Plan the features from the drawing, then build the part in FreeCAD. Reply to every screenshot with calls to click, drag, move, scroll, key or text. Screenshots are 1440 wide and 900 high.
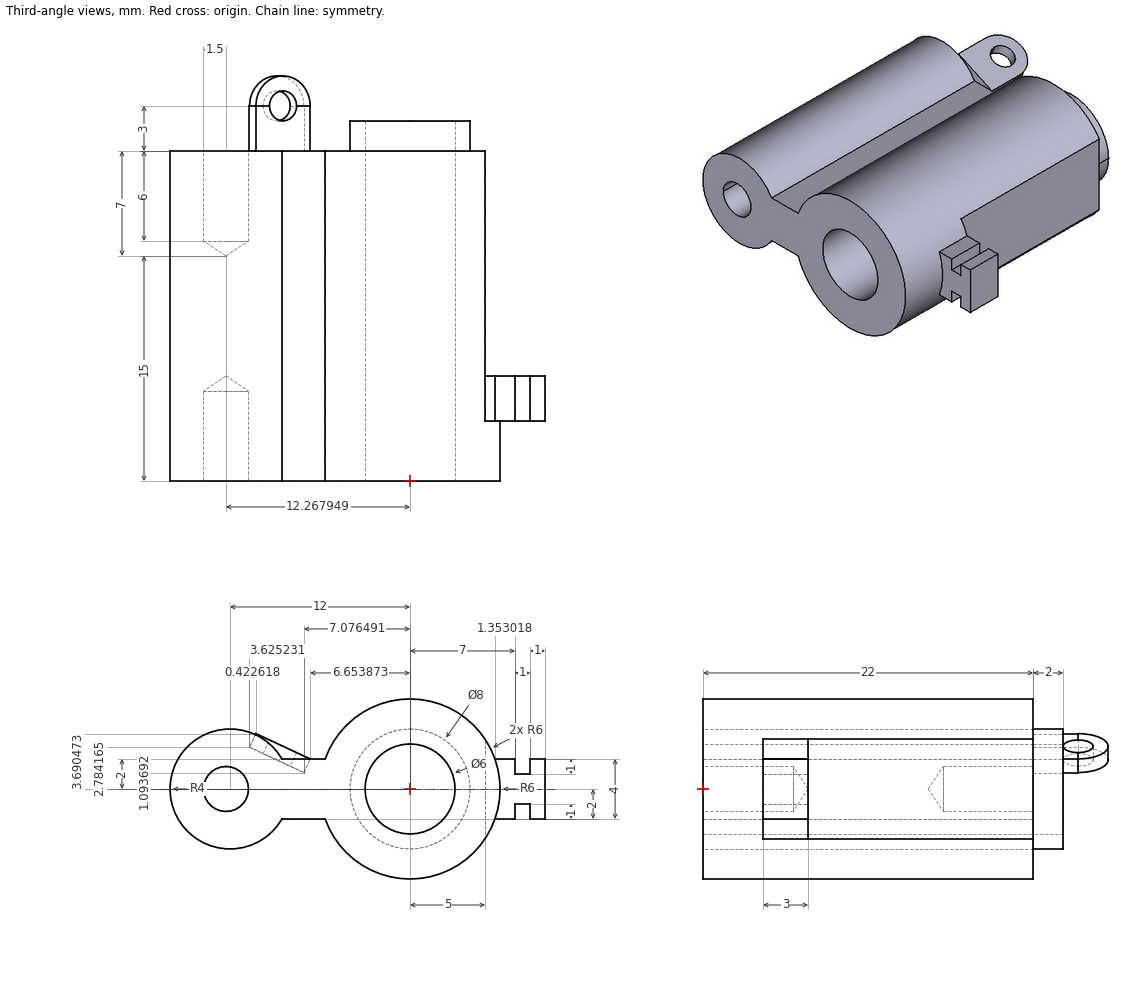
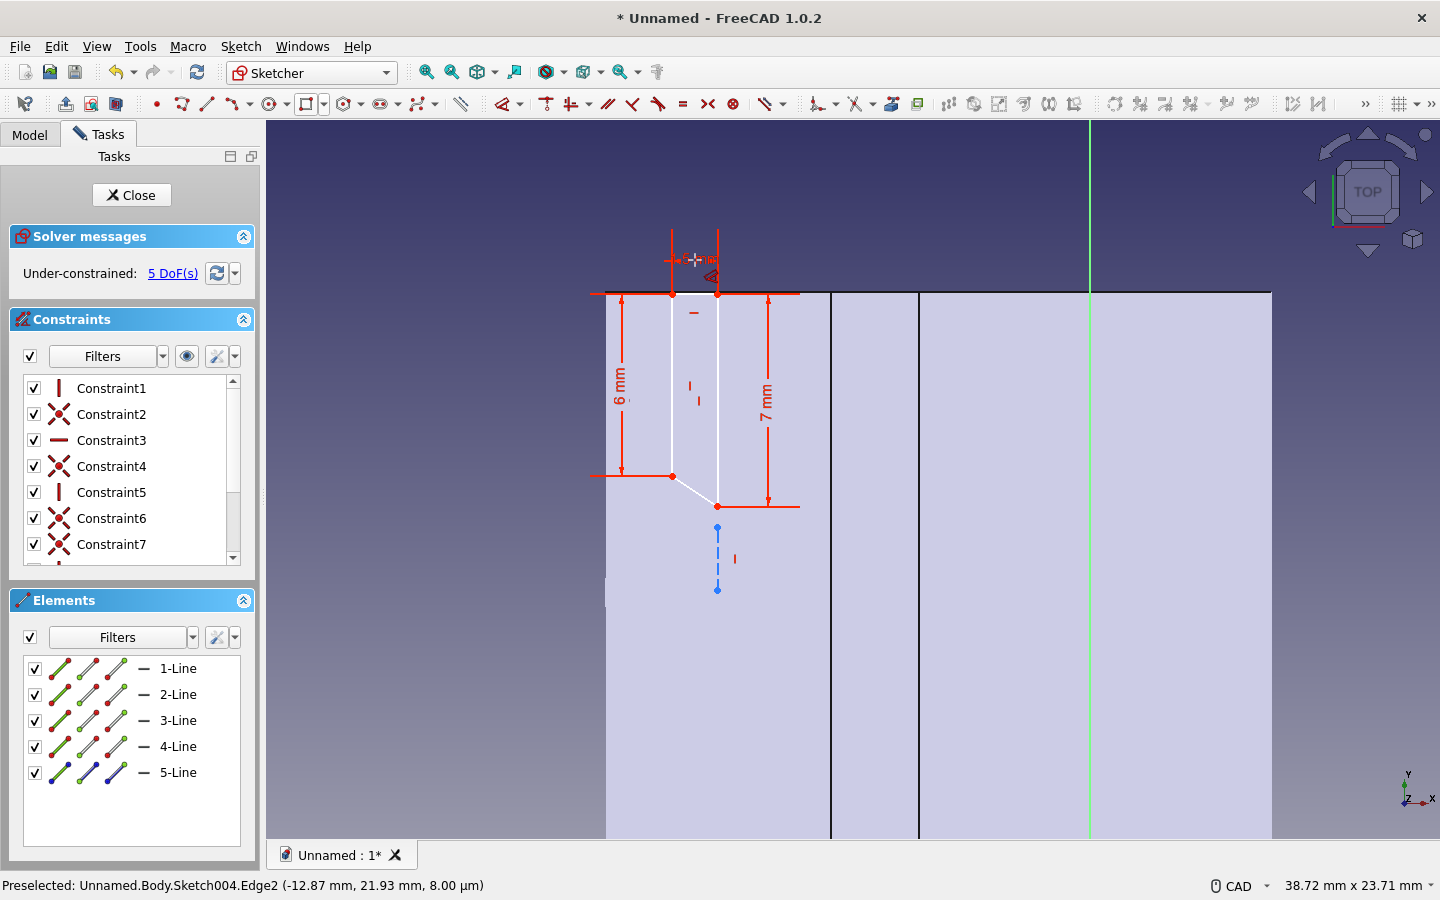
click(718, 507)
click(1124, 659)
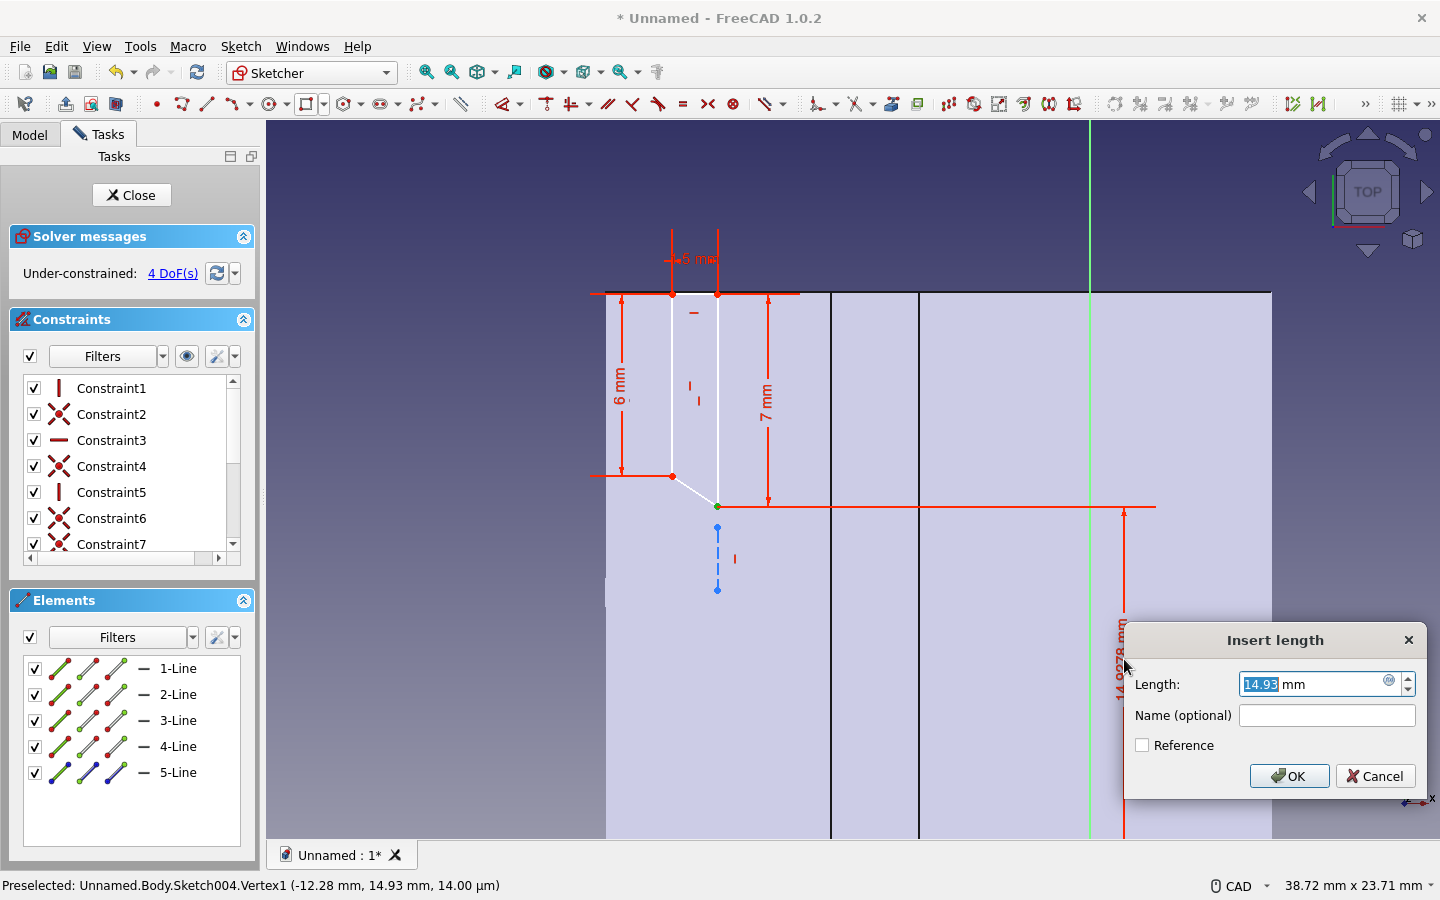
text(15)
key(Return)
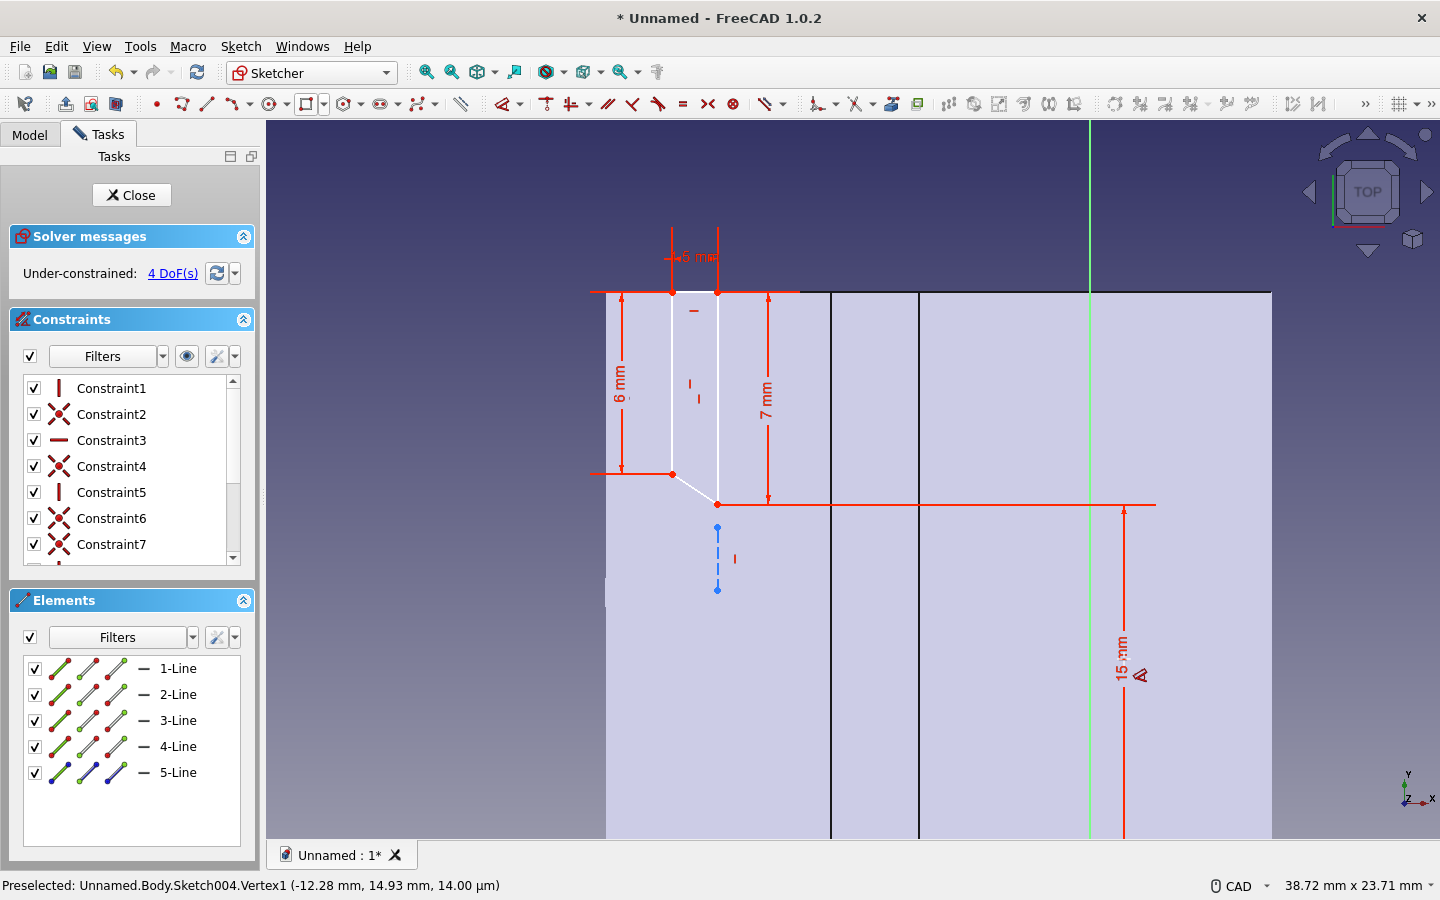
click(718, 505)
click(904, 471)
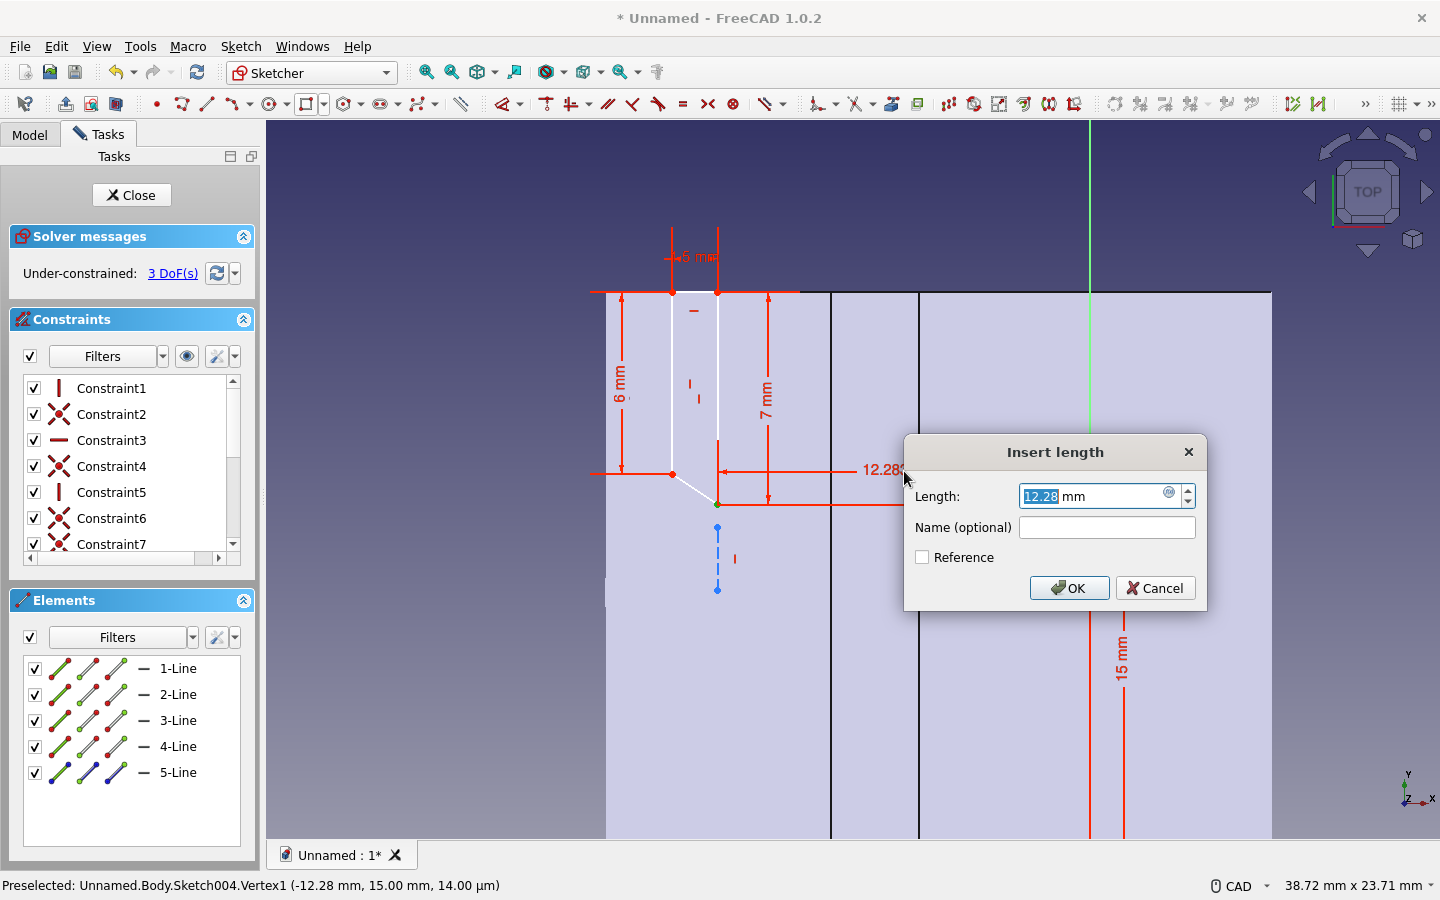
text(12.267949)
key(Return)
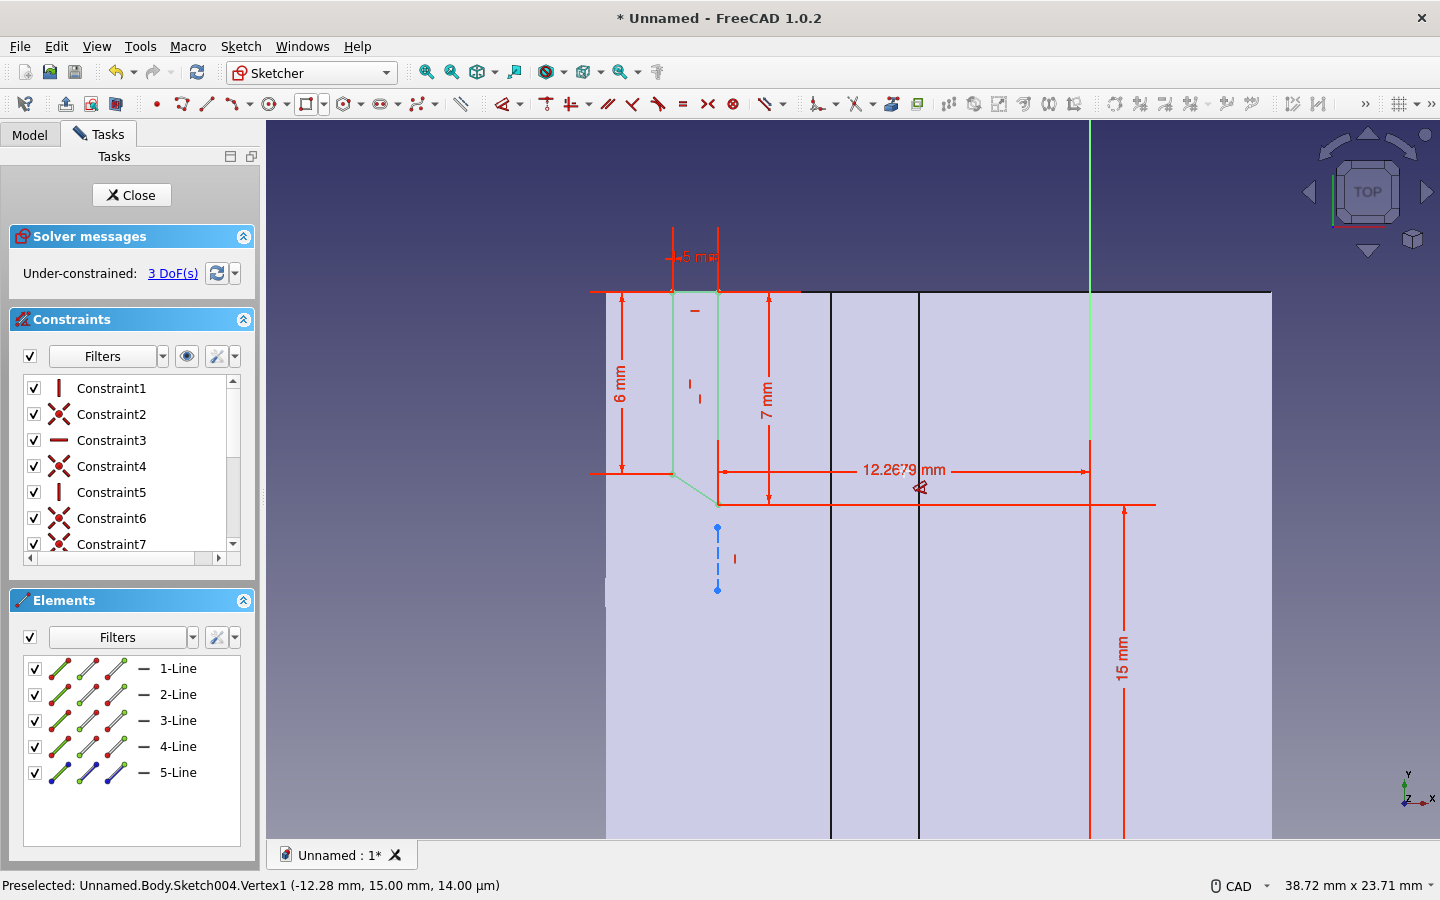
click(718, 528)
click(904, 494)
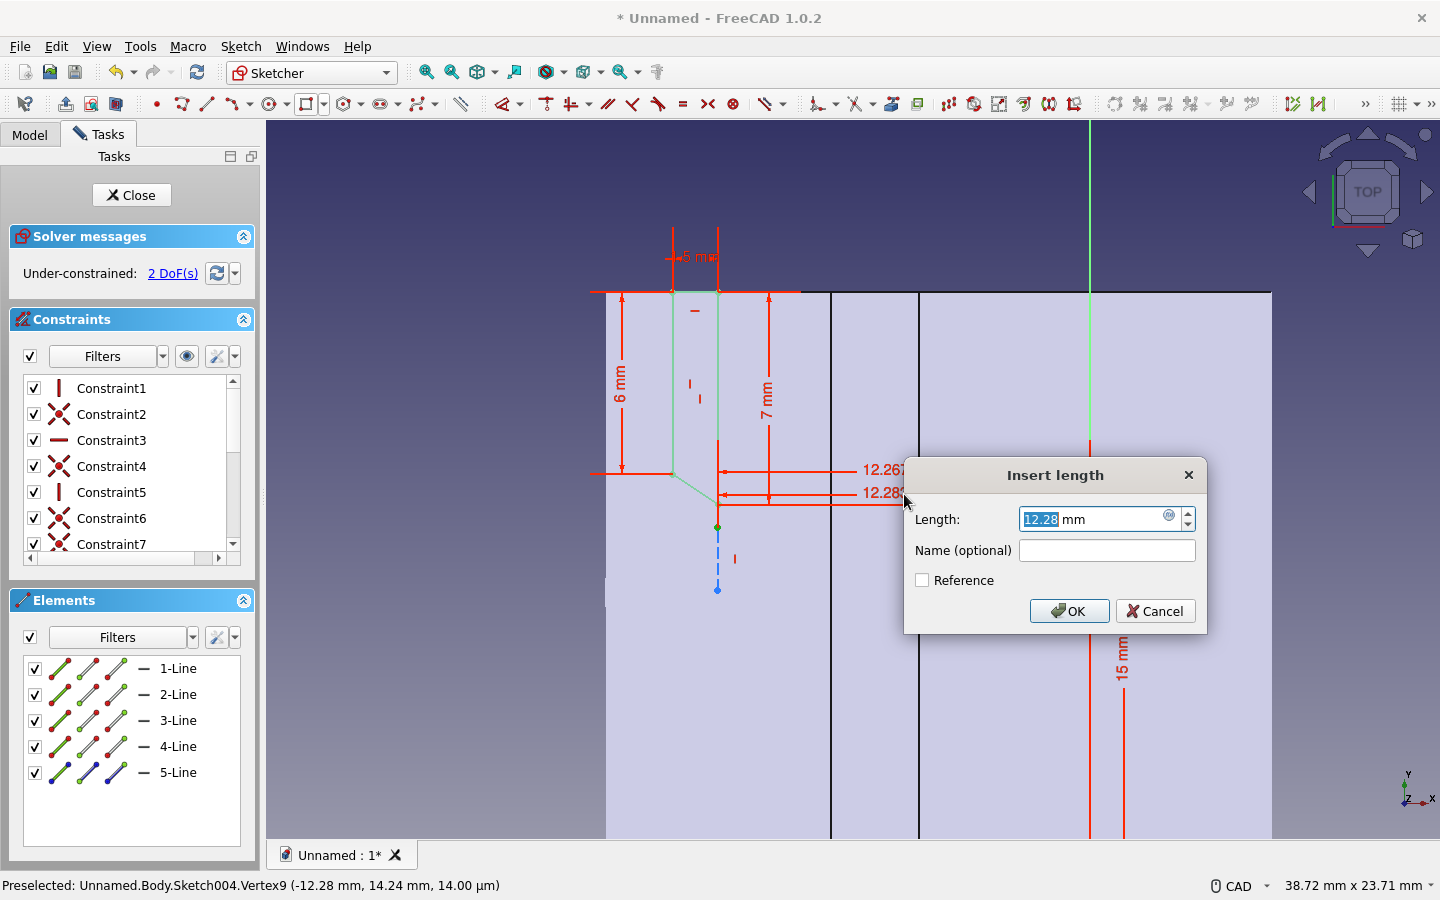
text(12.267949)
key(Return)
key(Escape)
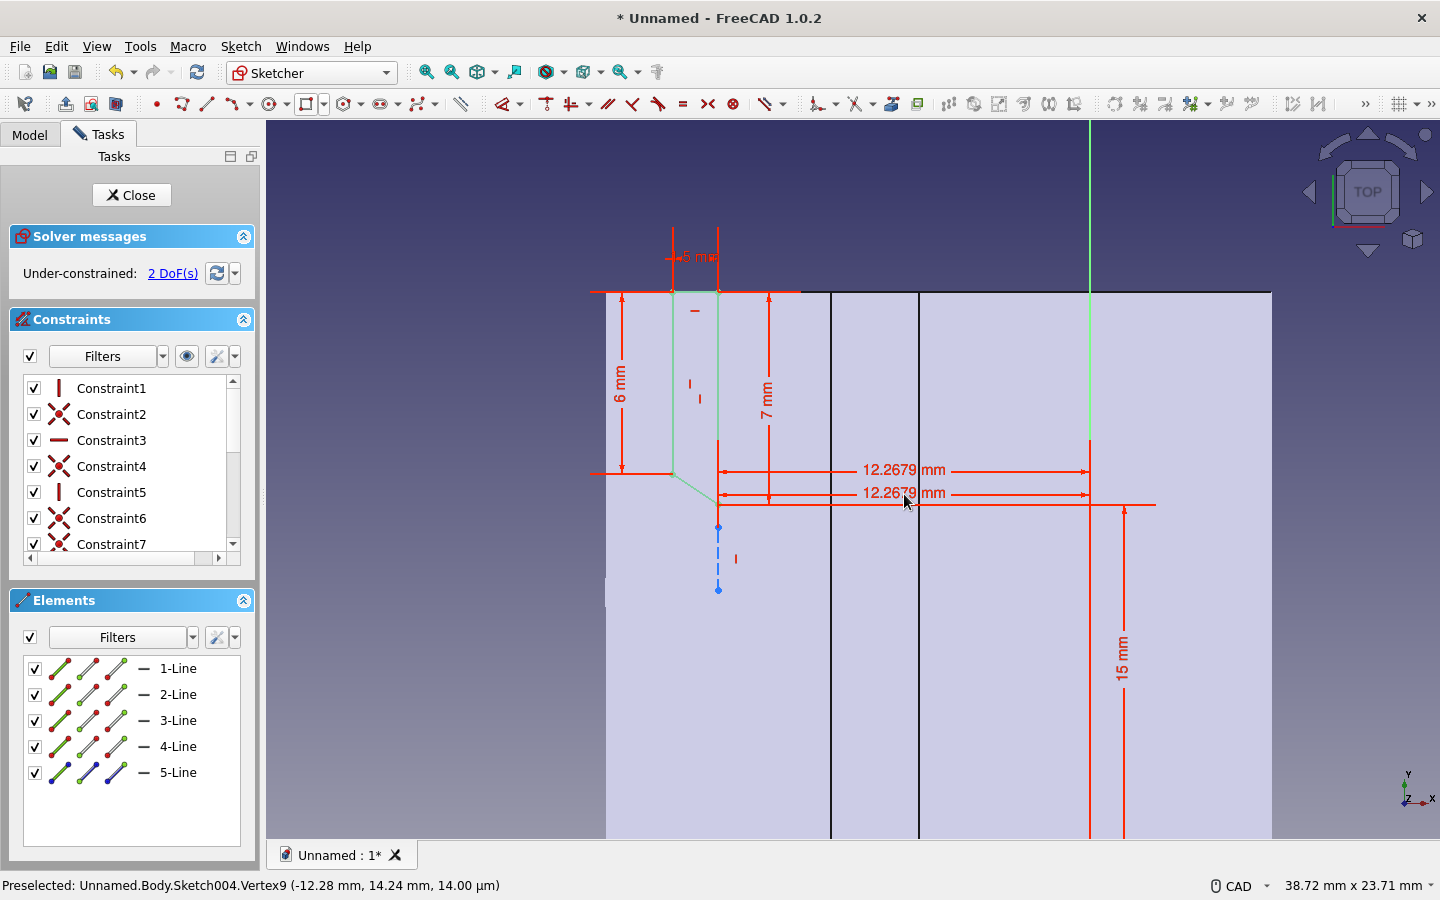
click(132, 195)